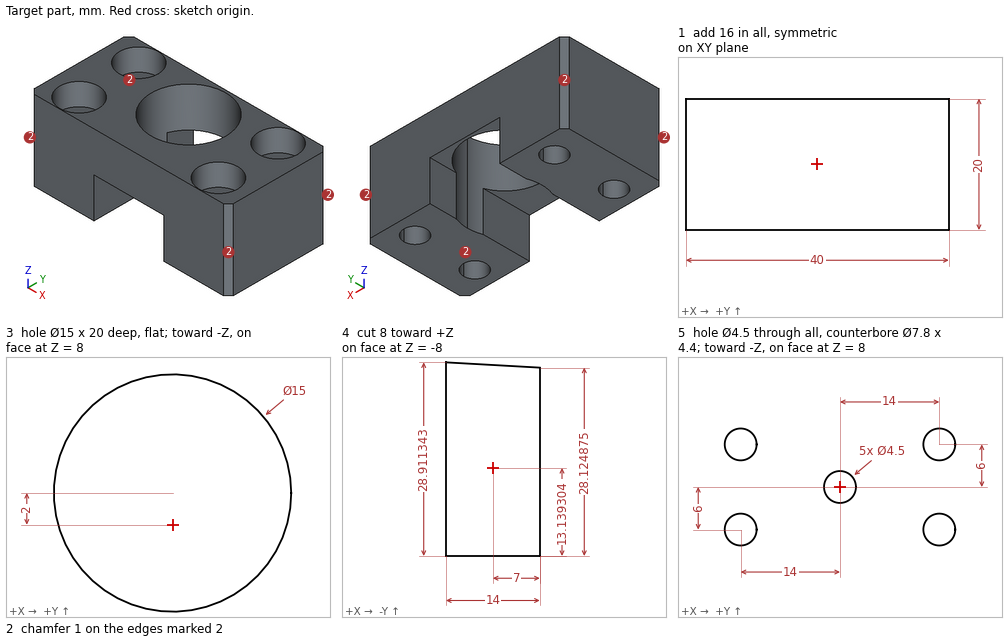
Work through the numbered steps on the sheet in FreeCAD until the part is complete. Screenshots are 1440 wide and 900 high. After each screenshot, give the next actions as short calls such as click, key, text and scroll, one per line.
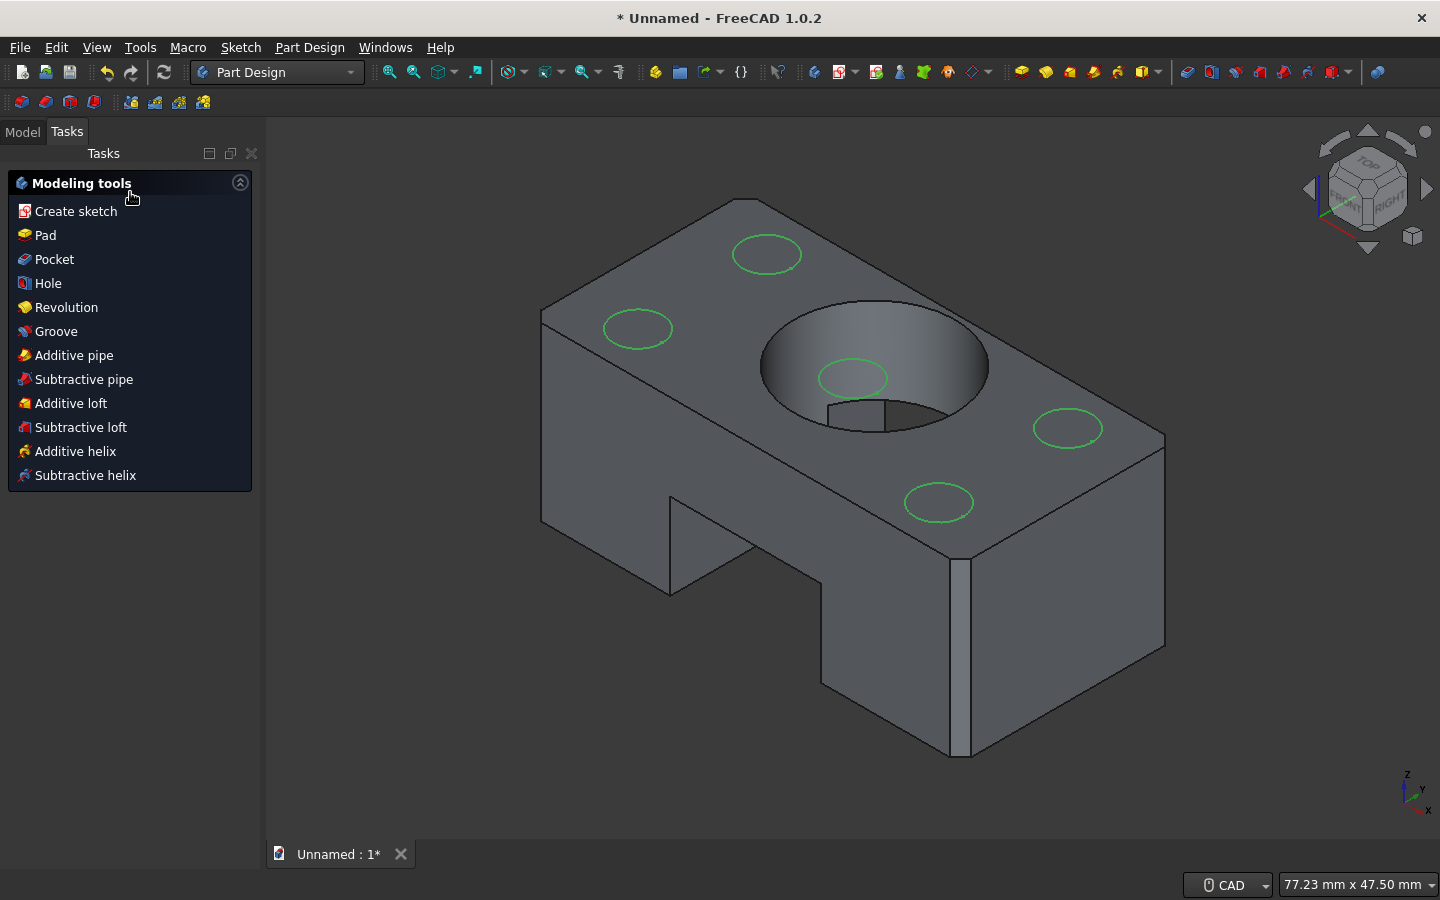
click(1212, 72)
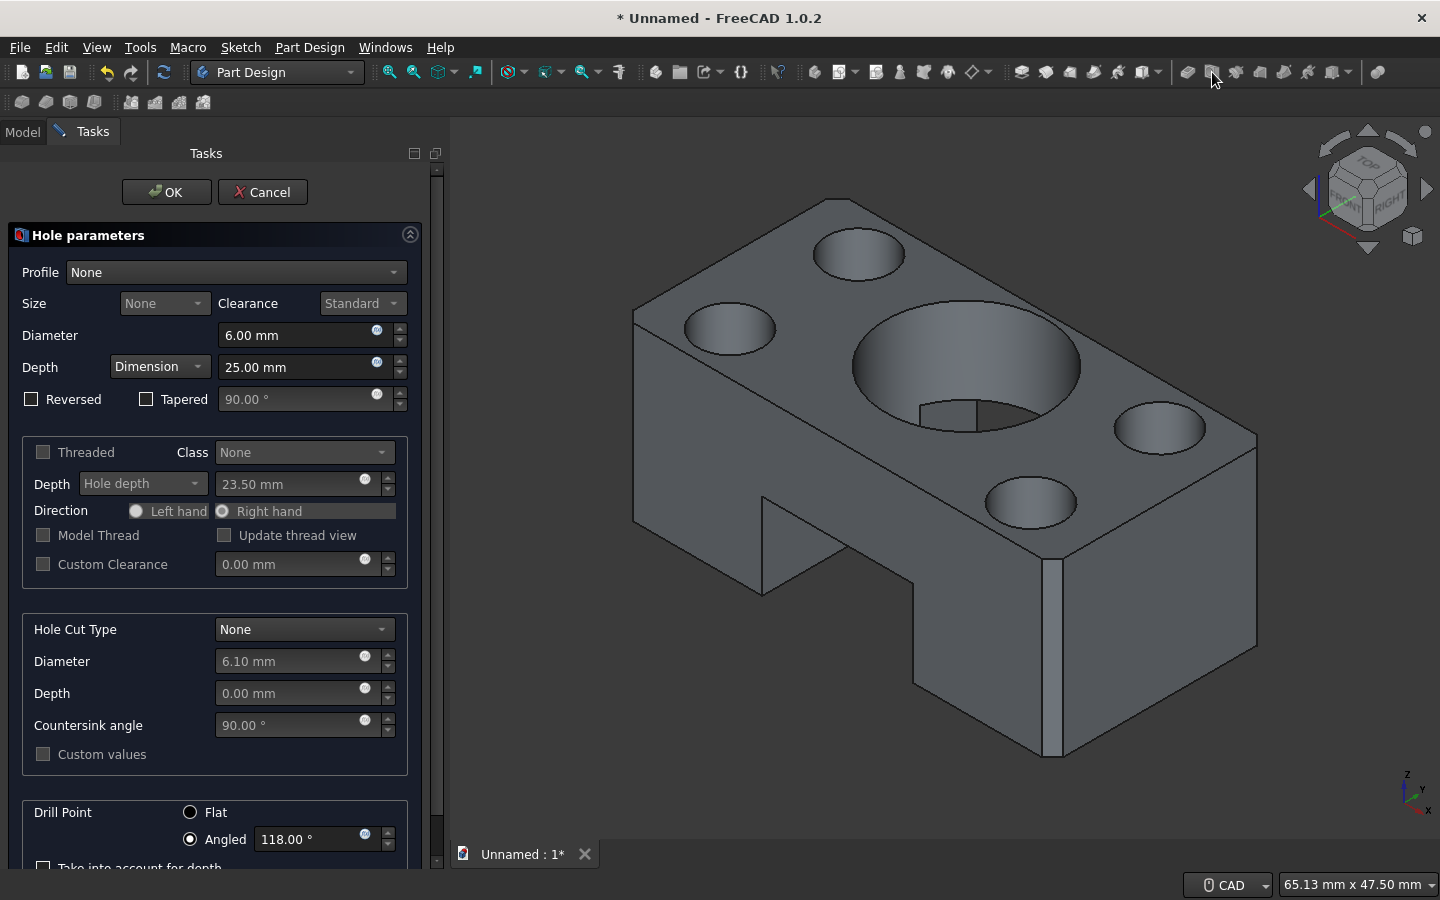
triple_click(305, 335)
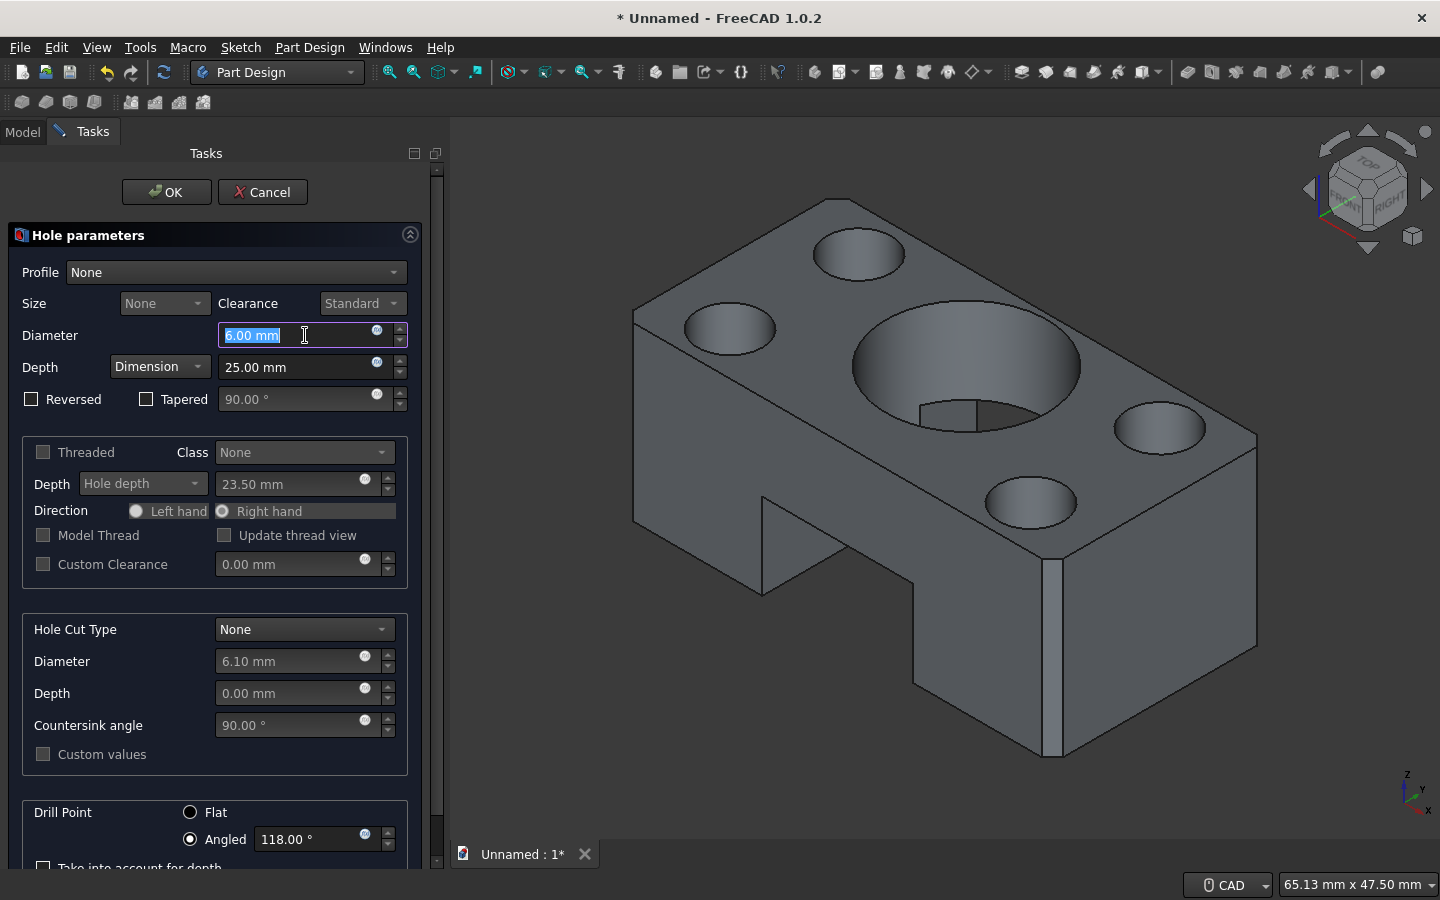
text(4.5)
key(Tab)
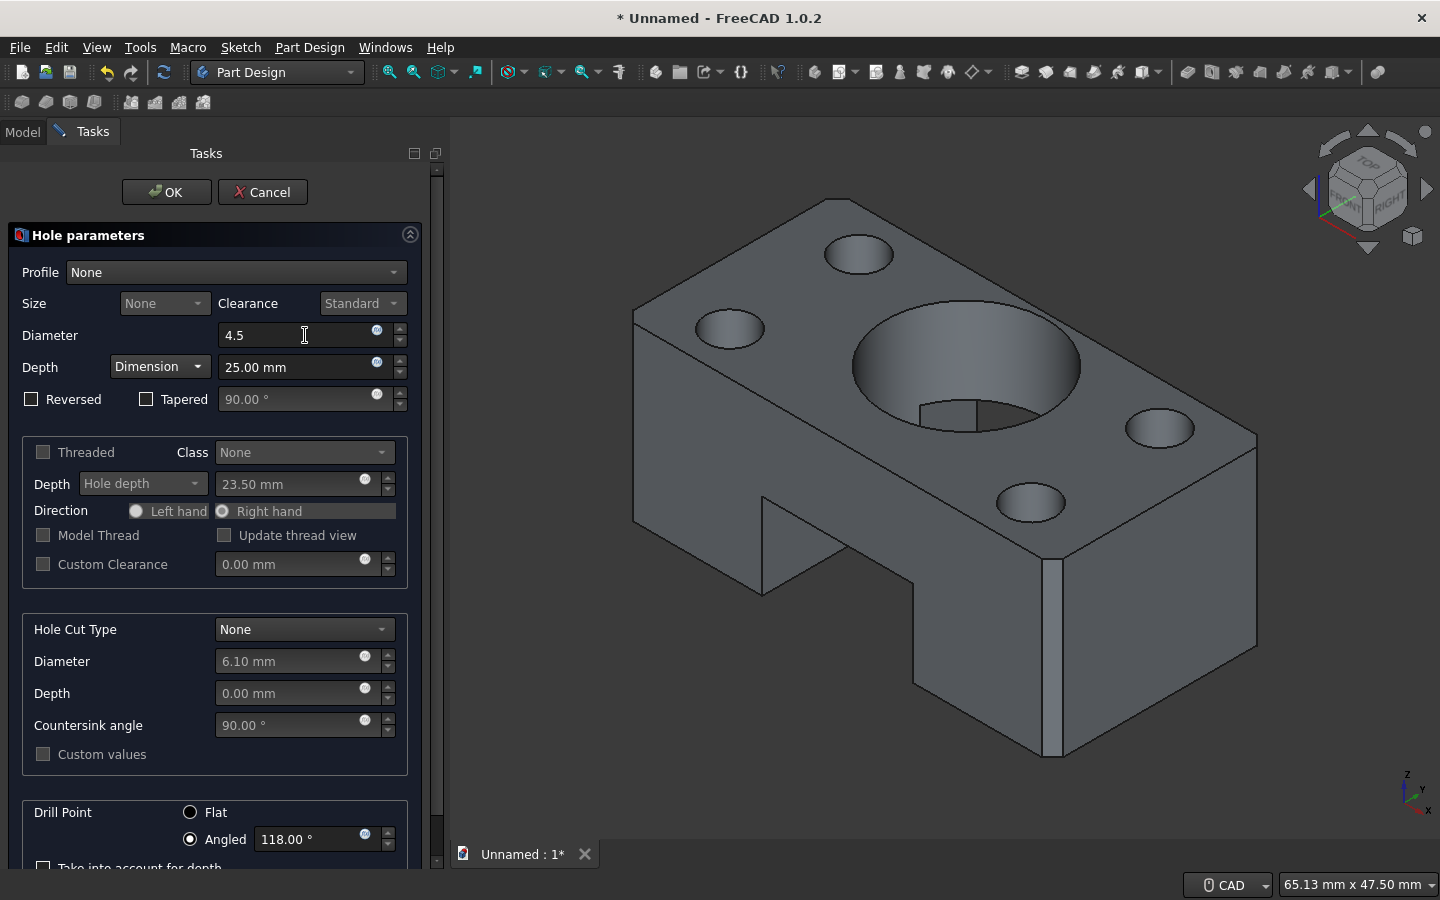
click(161, 366)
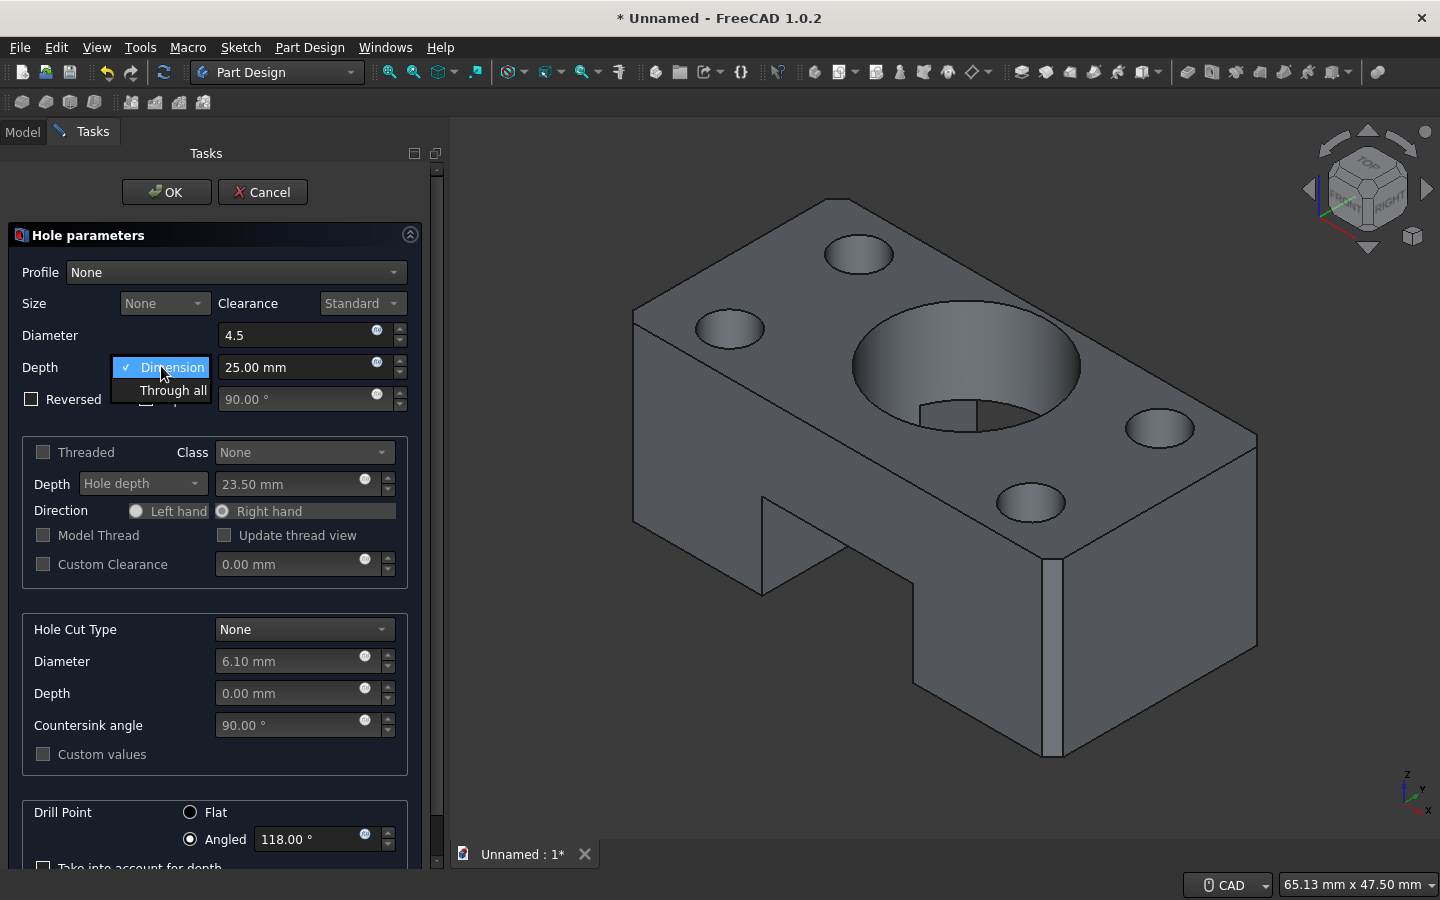
click(160, 390)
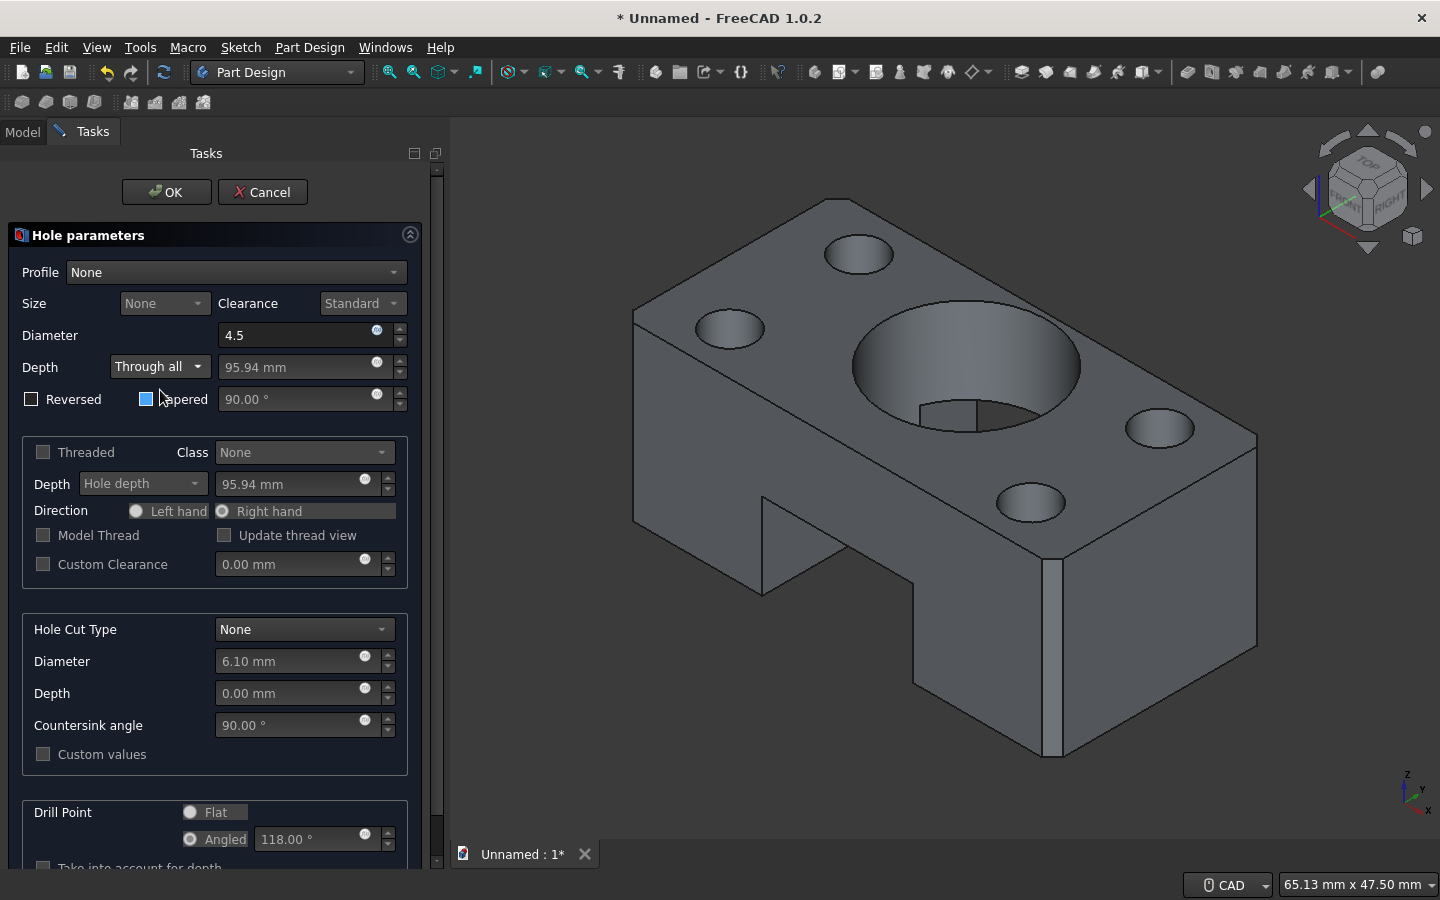
click(306, 630)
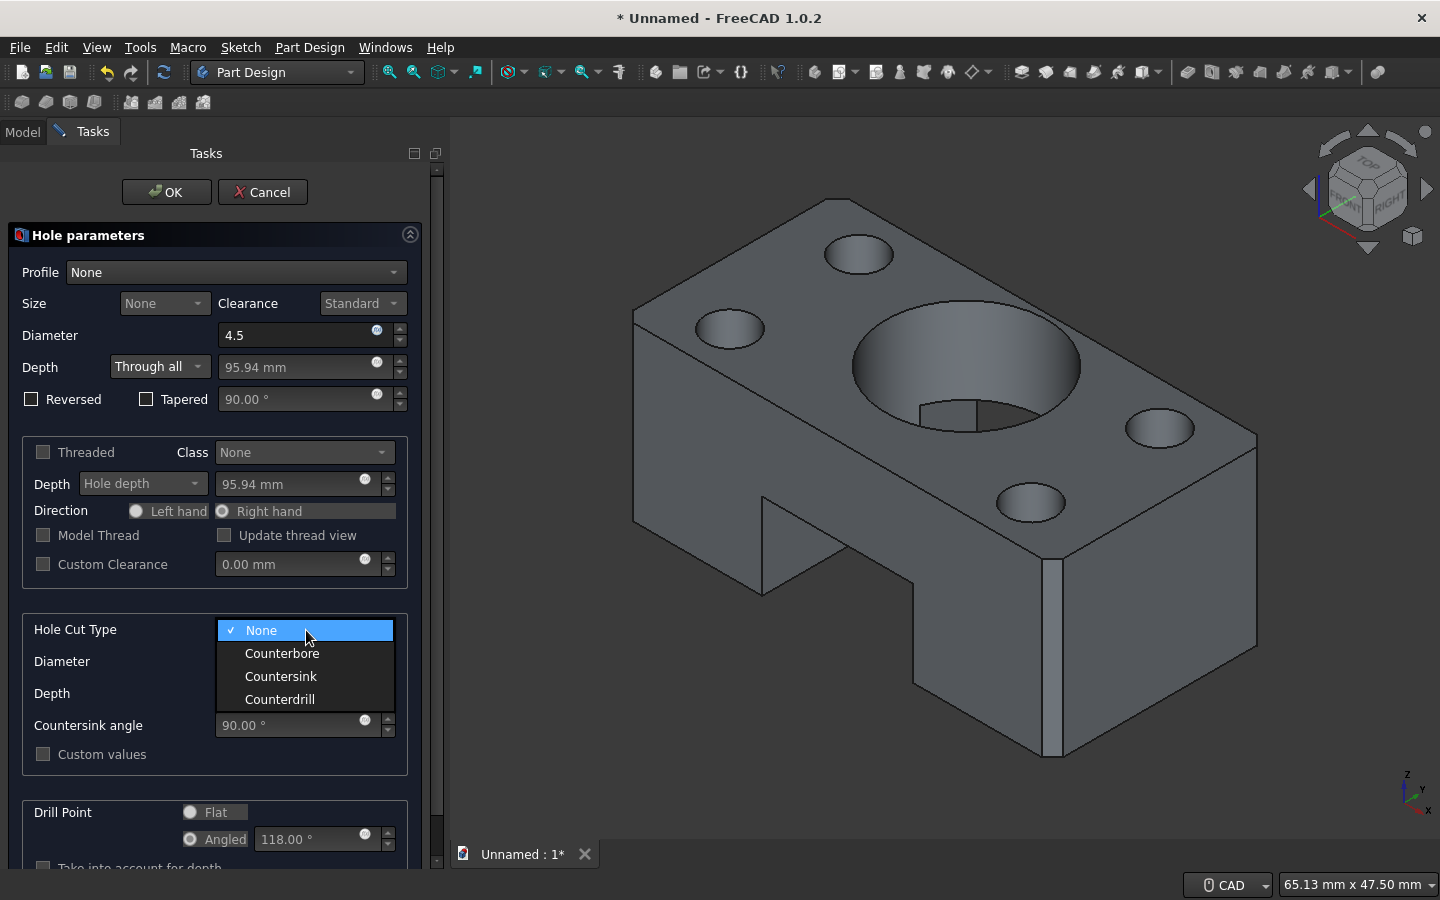
click(304, 654)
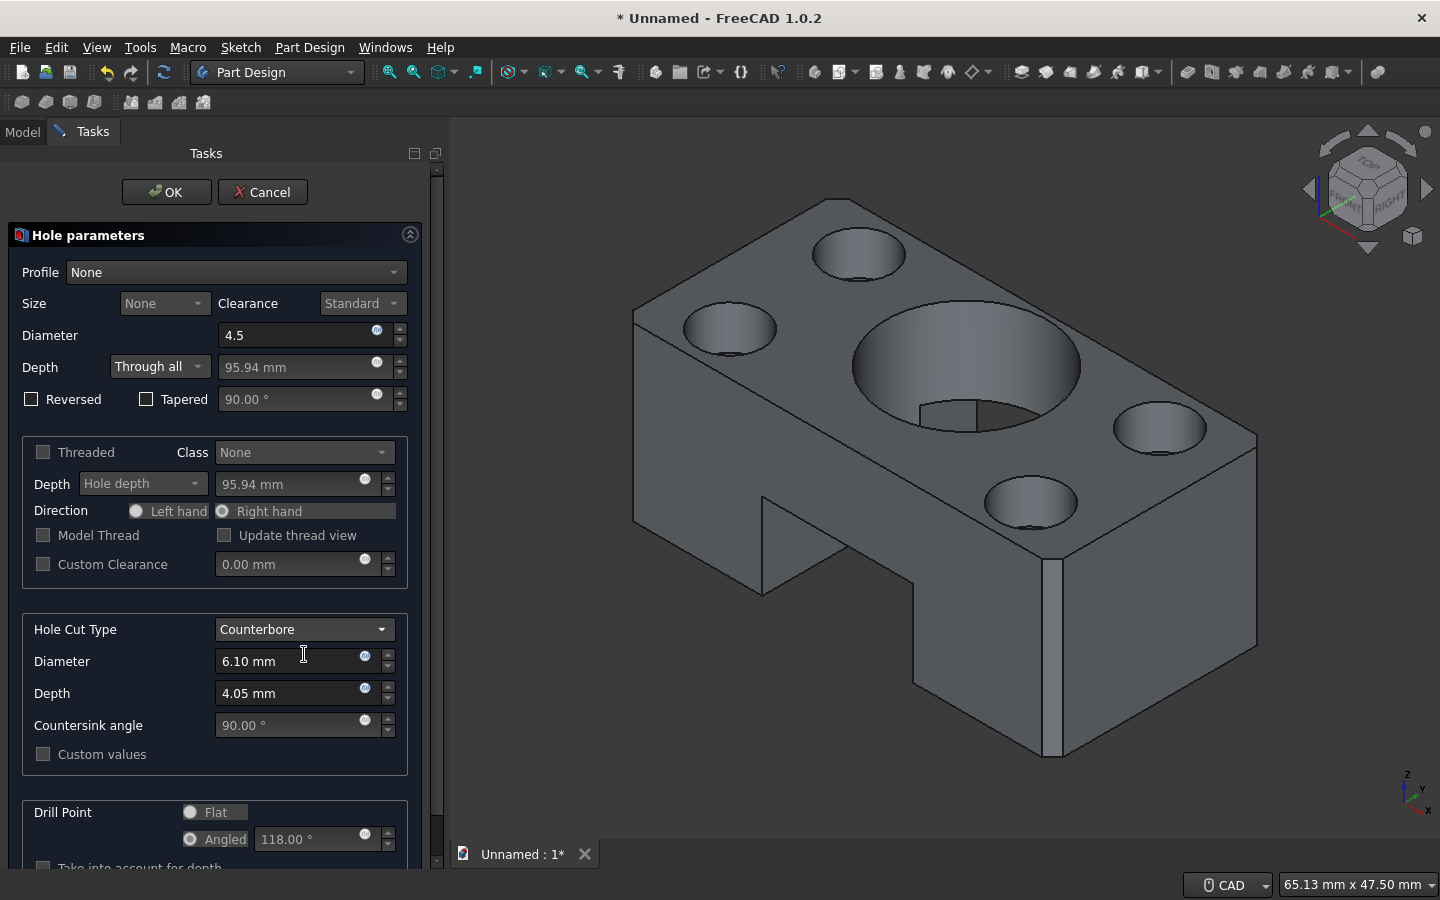
triple_click(298, 661)